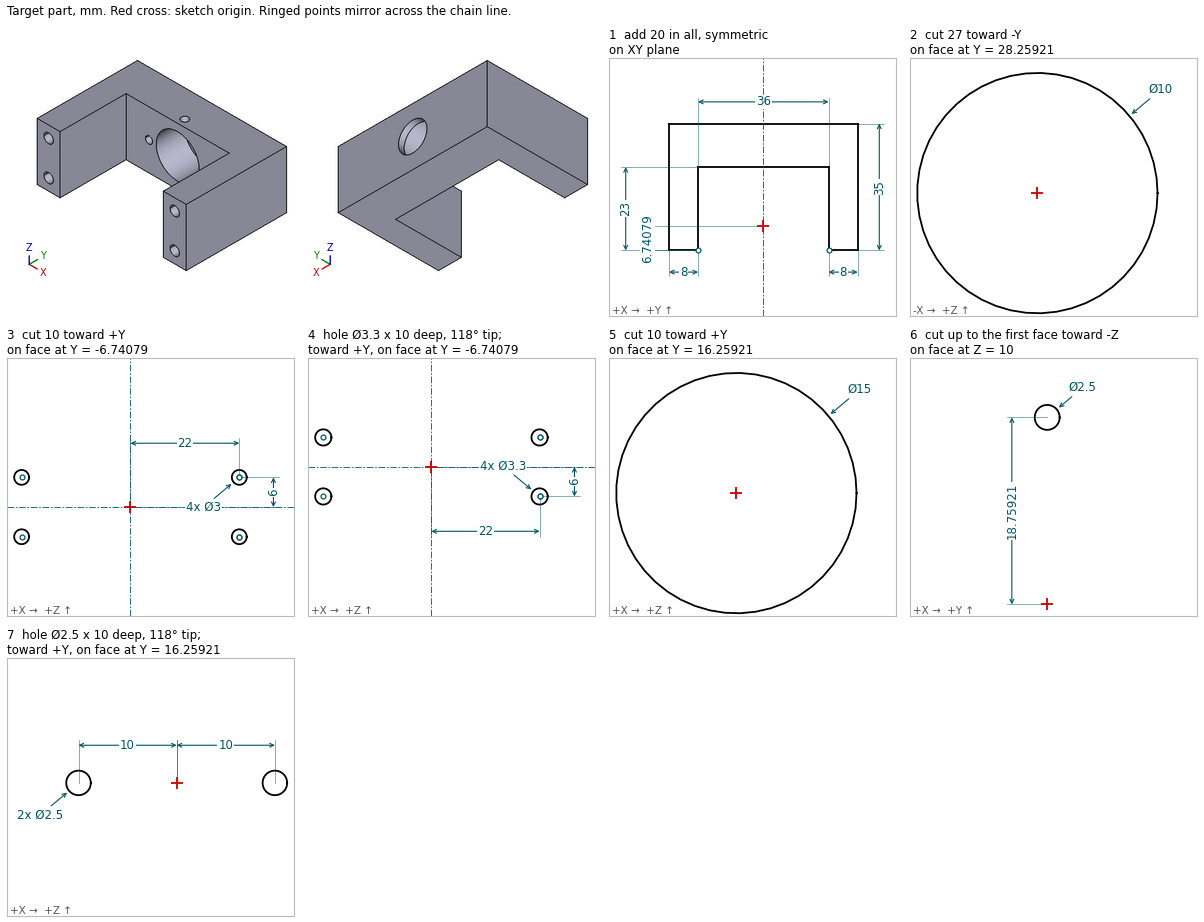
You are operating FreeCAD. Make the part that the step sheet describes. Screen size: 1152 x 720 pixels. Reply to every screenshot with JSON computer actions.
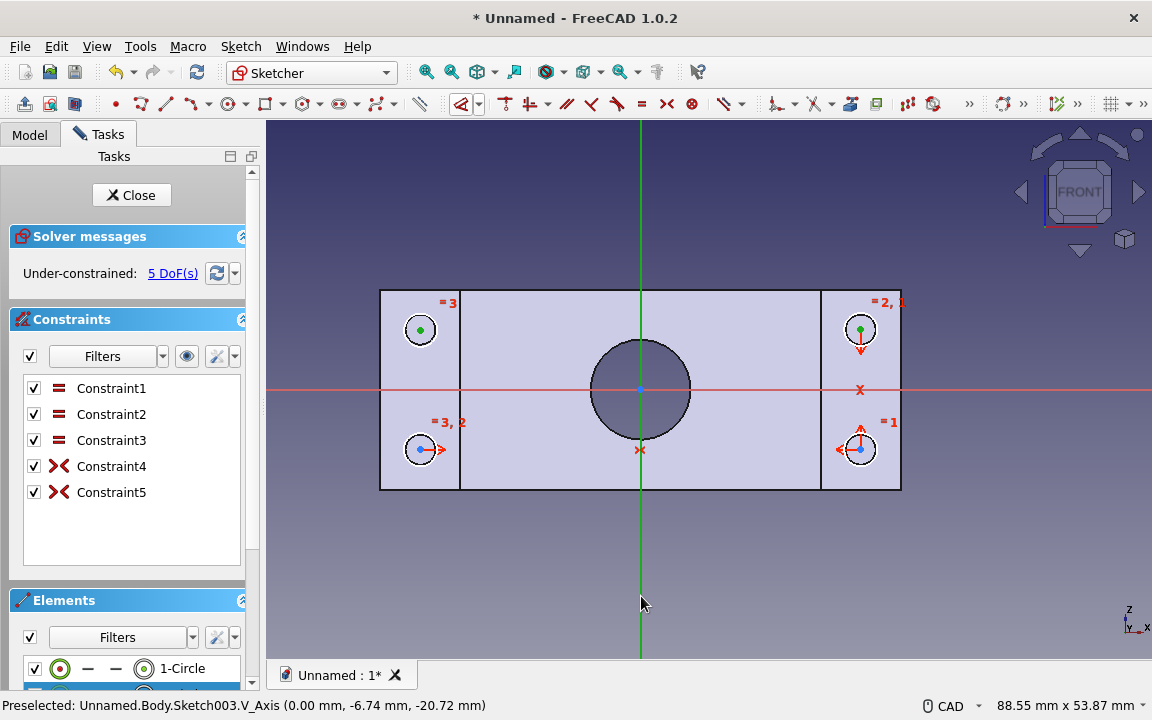
{"action": "key", "text": "s"}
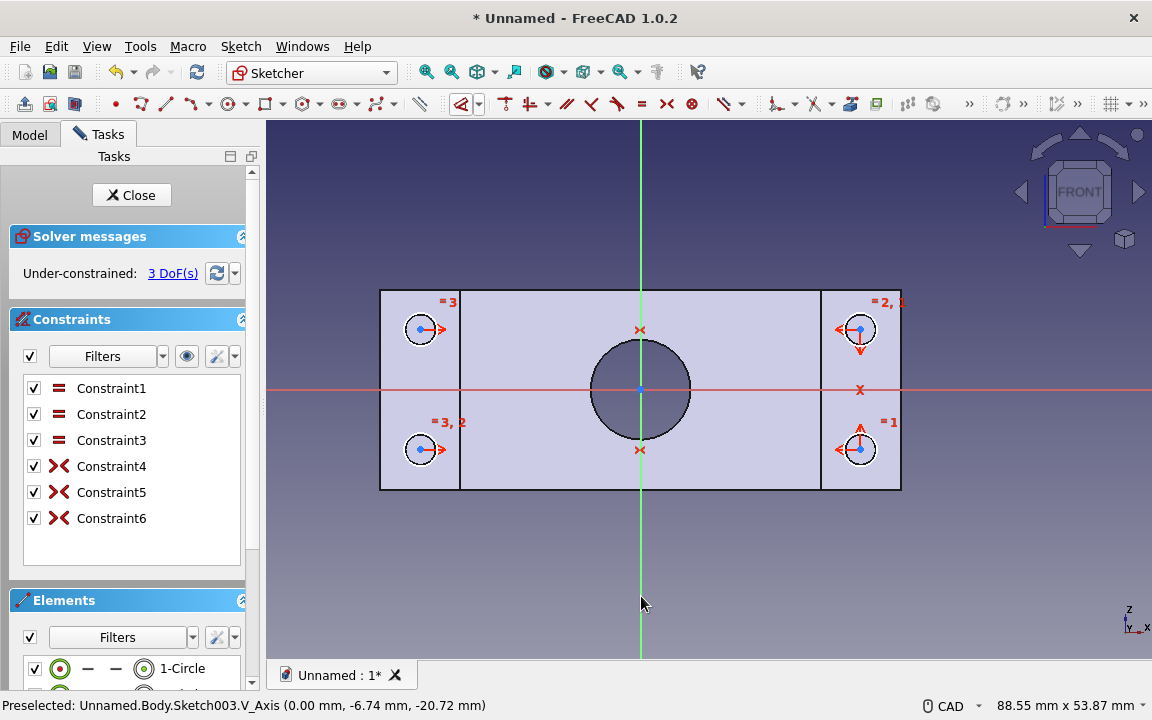
{"action": "left_click", "coordinate": [872, 438]}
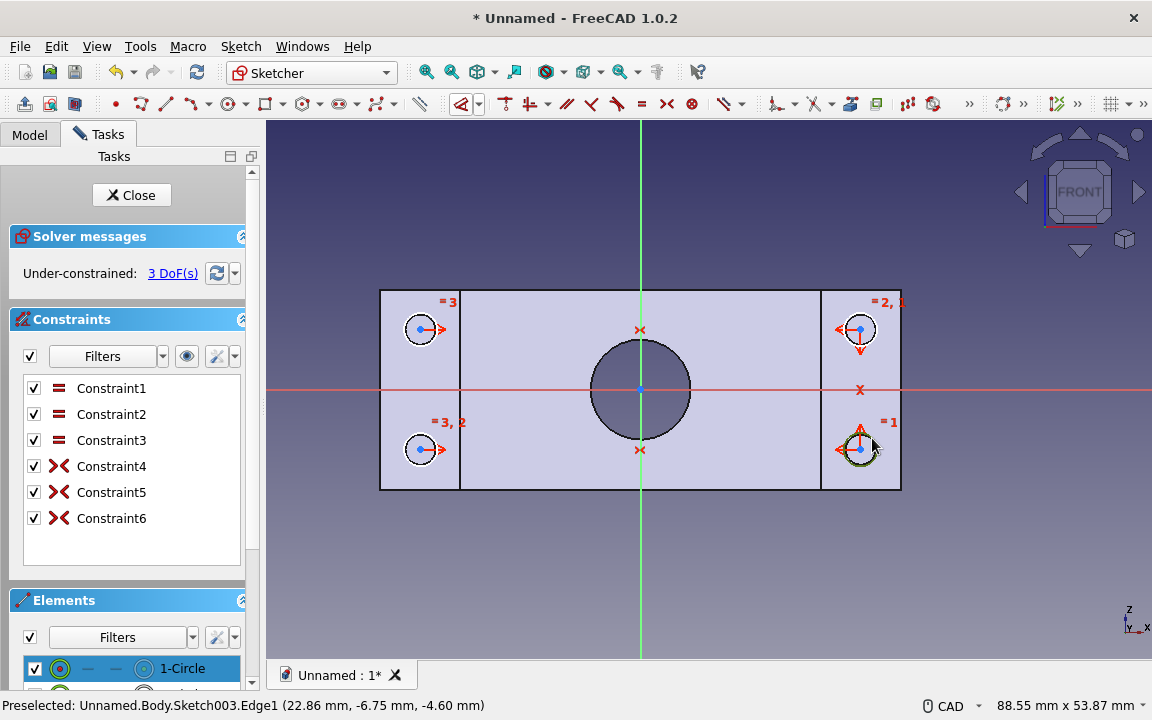
{"action": "key", "text": "k o"}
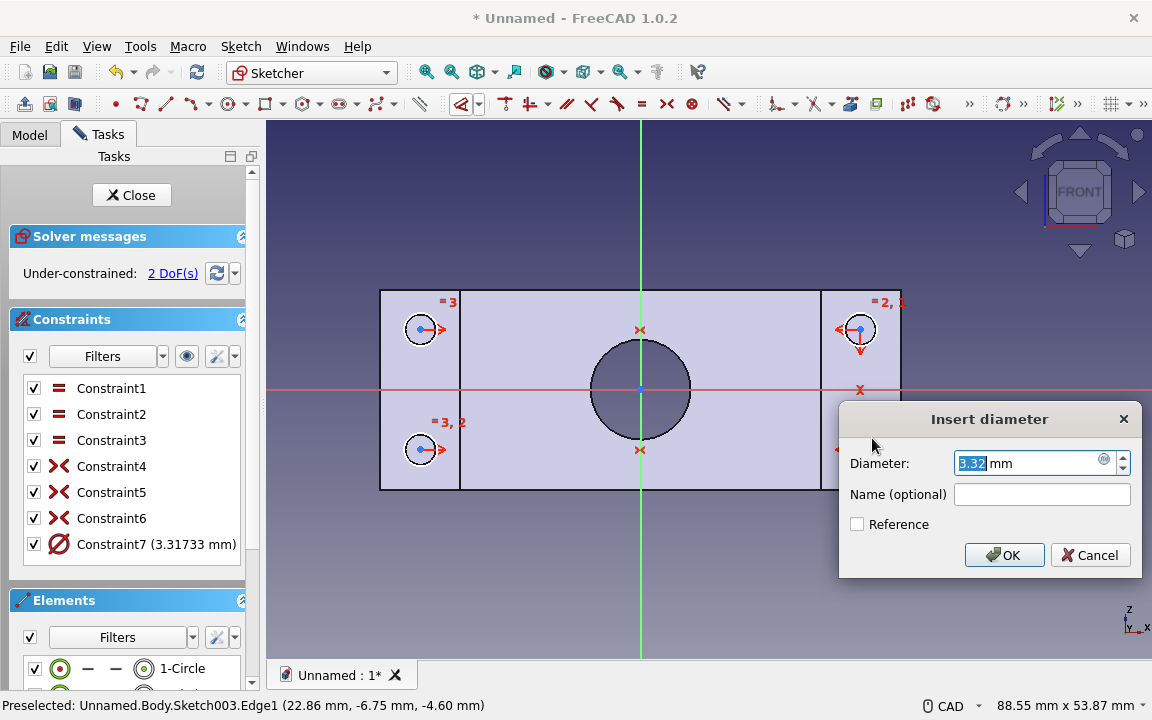
{"action": "type", "text": "3.3"}
{"action": "key", "text": "Return"}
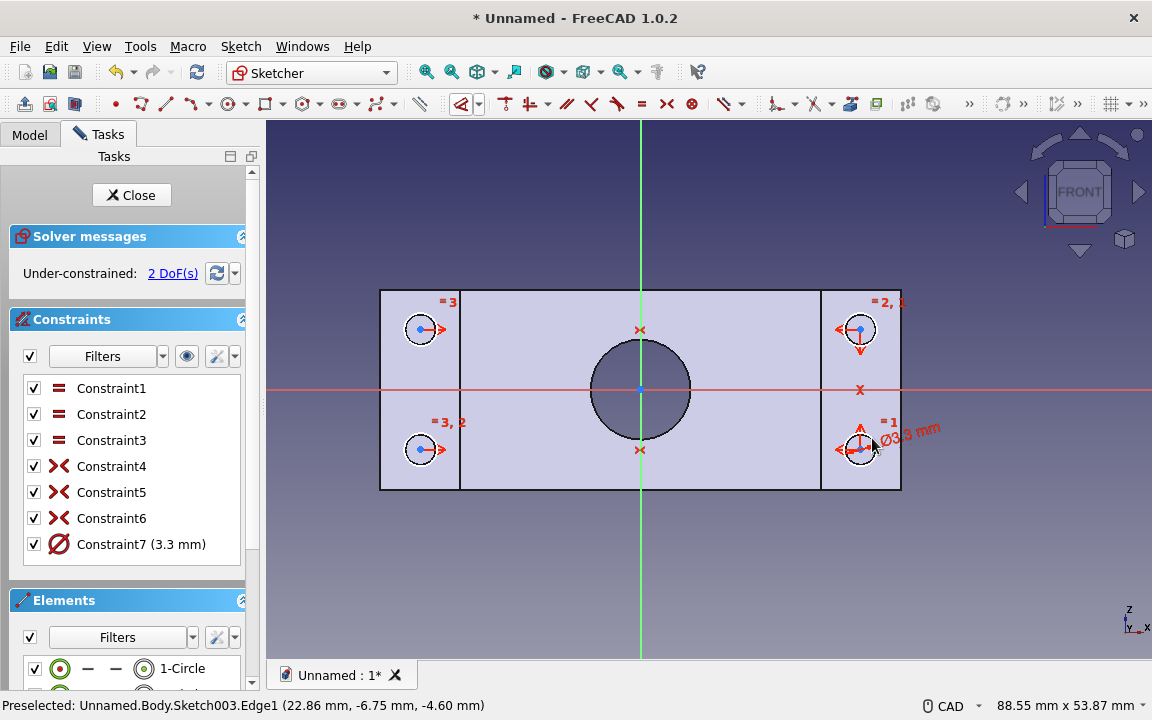
{"action": "left_click", "coordinate": [860, 450]}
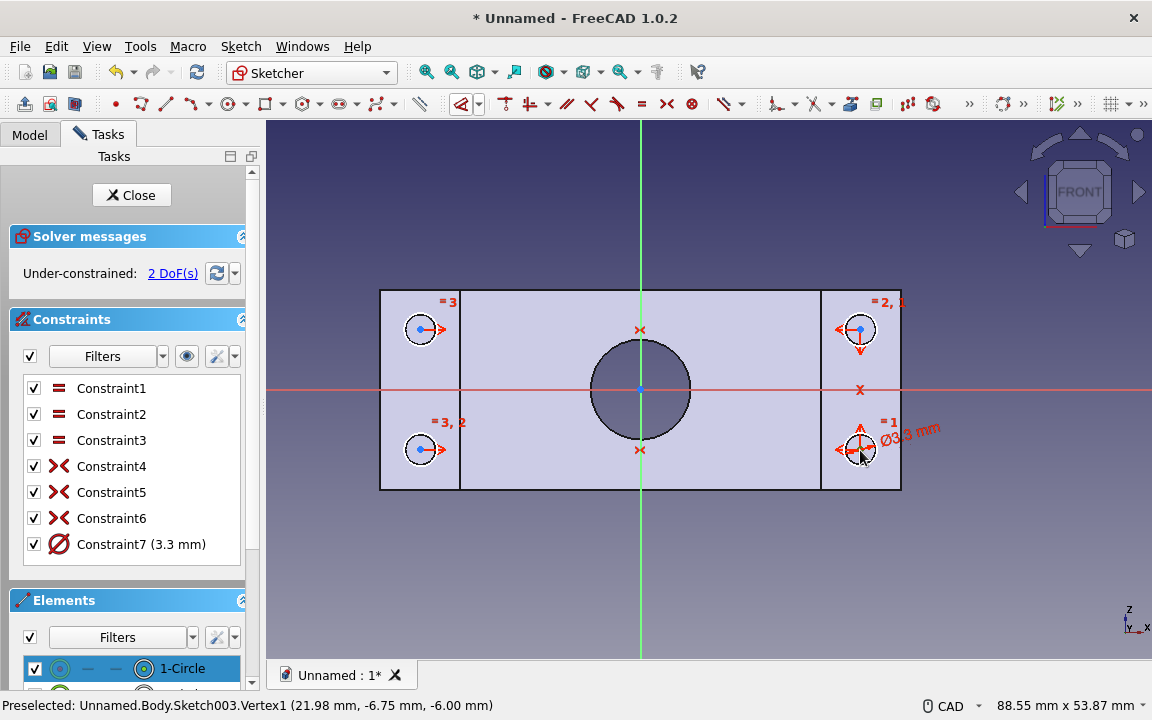
{"action": "key", "text": "i"}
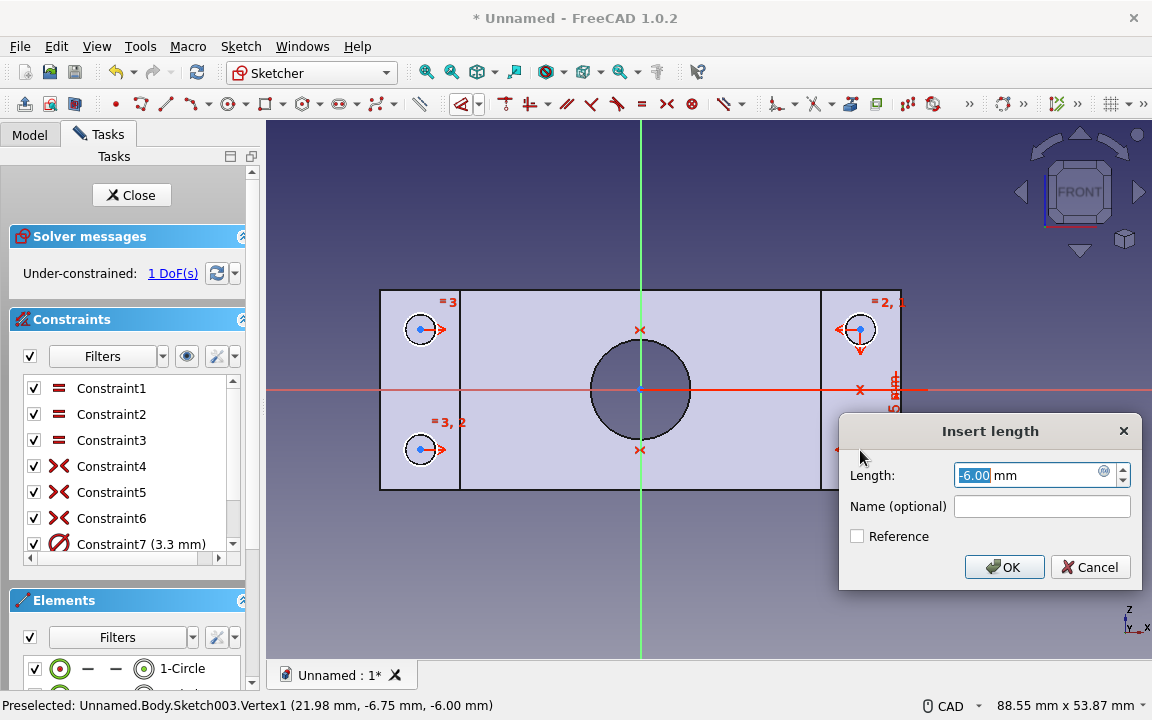
{"action": "type", "text": "-6"}
{"action": "key", "text": "Return"}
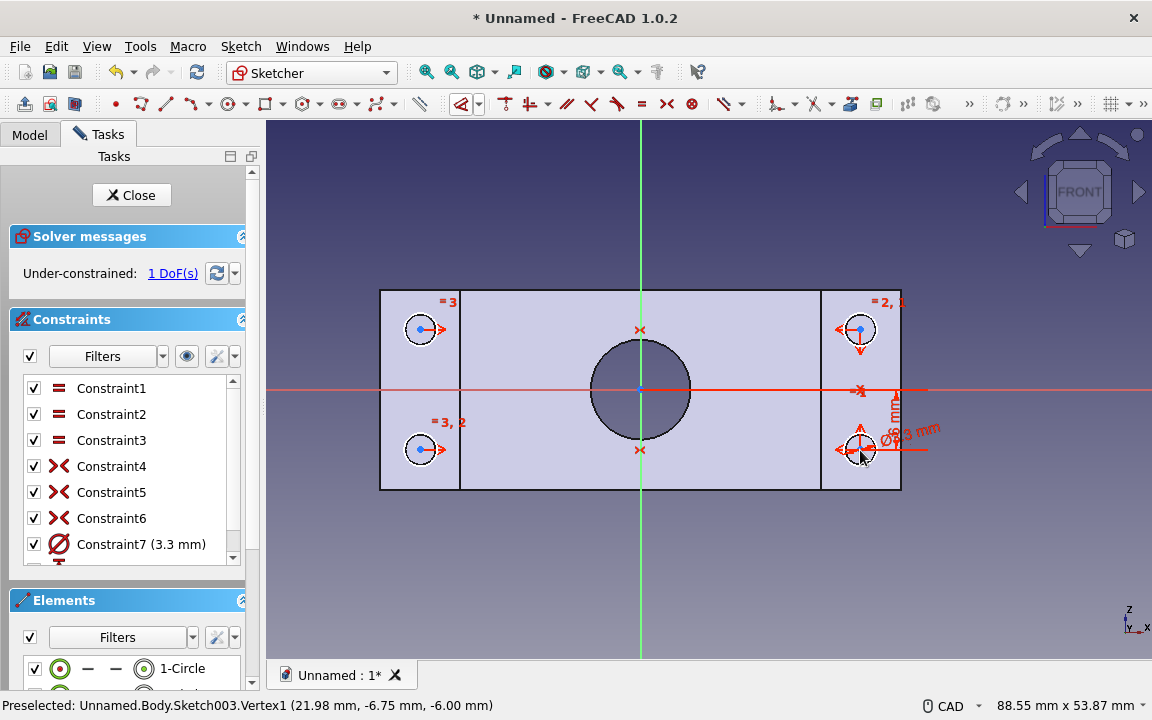
{"action": "left_click", "coordinate": [860, 450]}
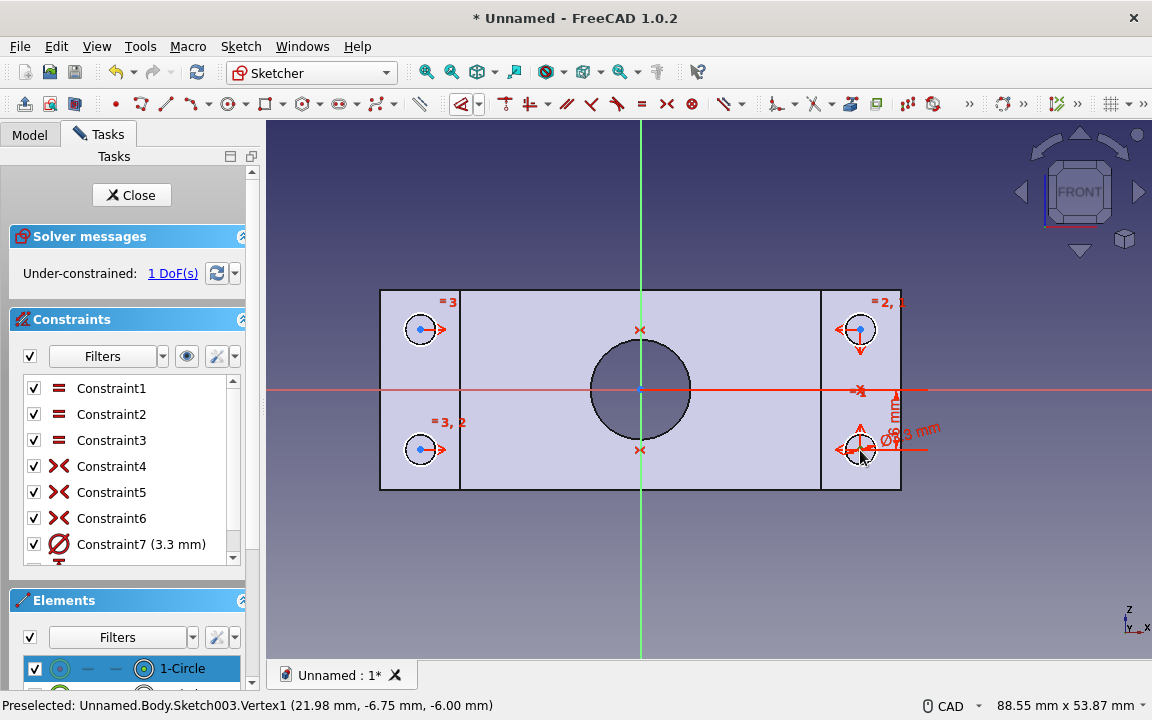
{"action": "key", "text": "l"}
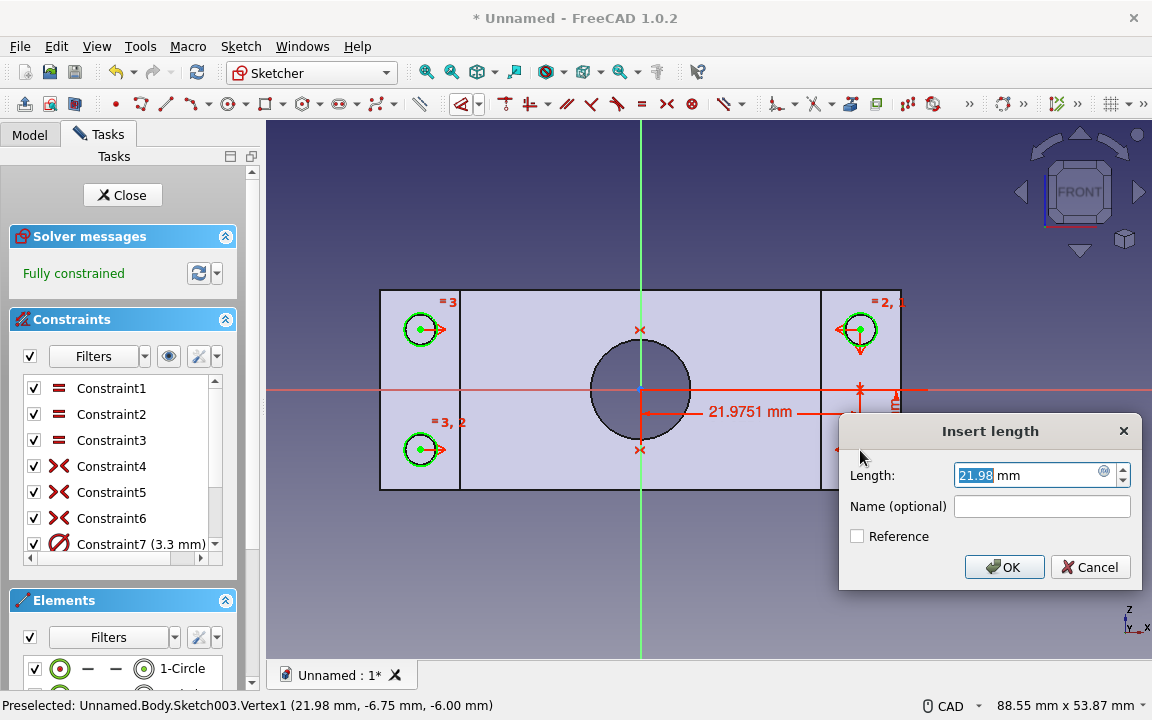
{"action": "type", "text": "22"}
{"action": "key", "text": "Return"}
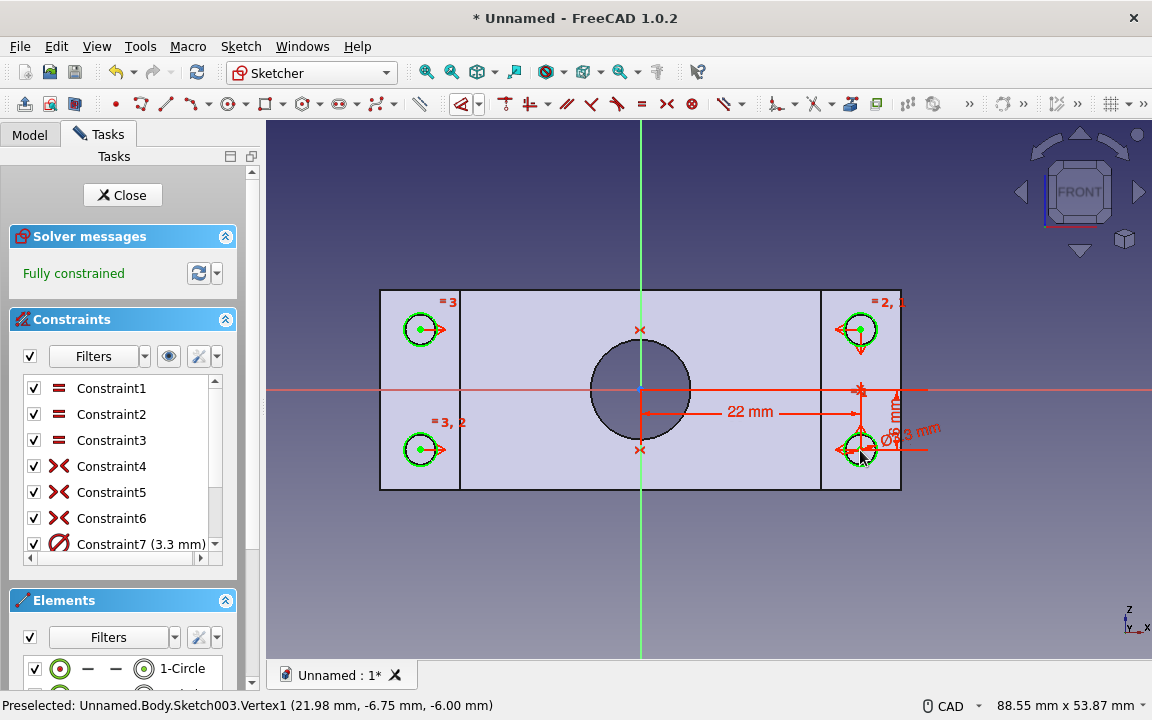
{"action": "left_click", "coordinate": [123, 195]}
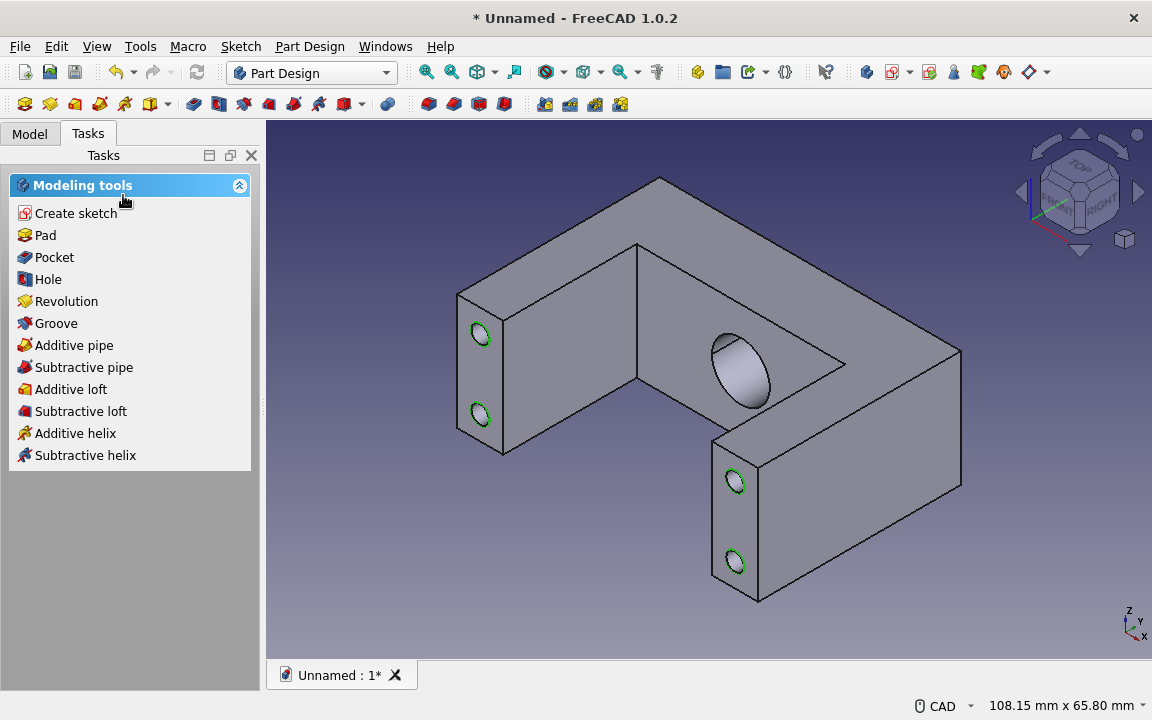
{"action": "left_click", "coordinate": [219, 104]}